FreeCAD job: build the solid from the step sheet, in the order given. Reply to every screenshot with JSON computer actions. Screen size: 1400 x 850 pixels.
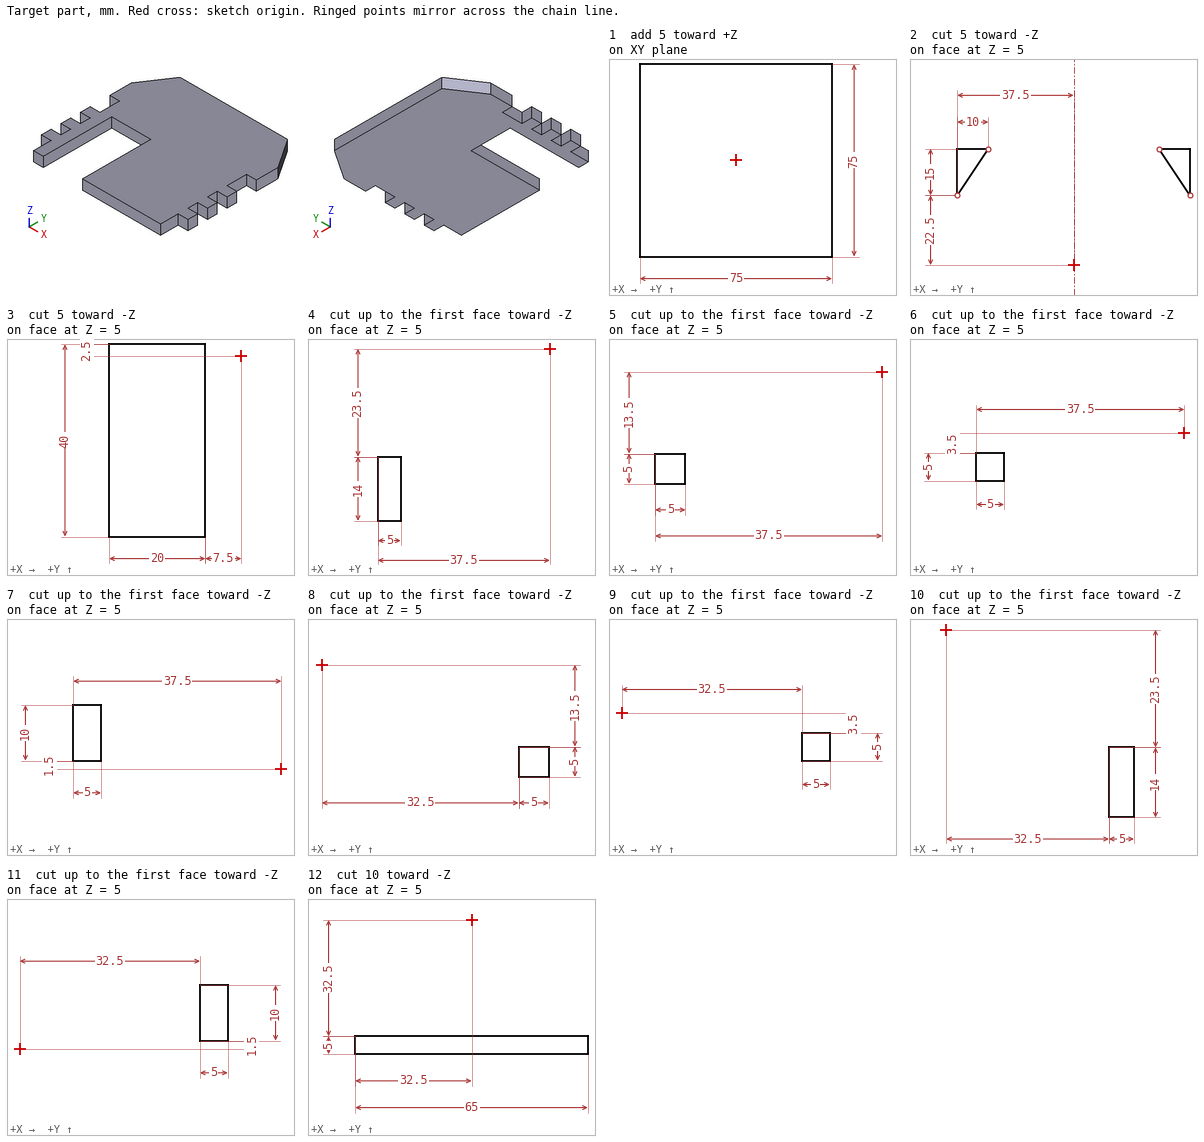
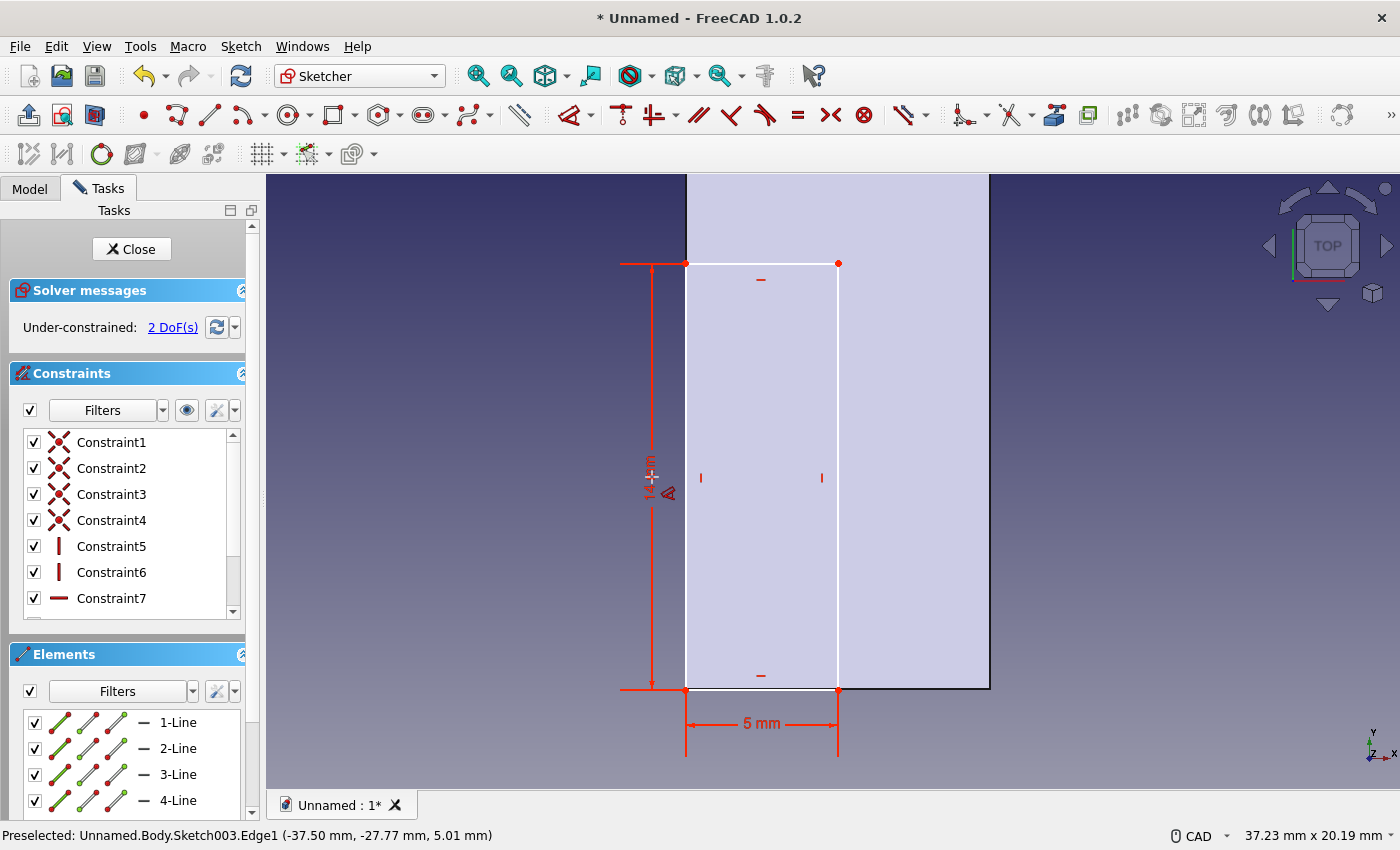
{"action": "left_click", "coordinate": [686, 264]}
{"action": "left_click", "coordinate": [960, 298]}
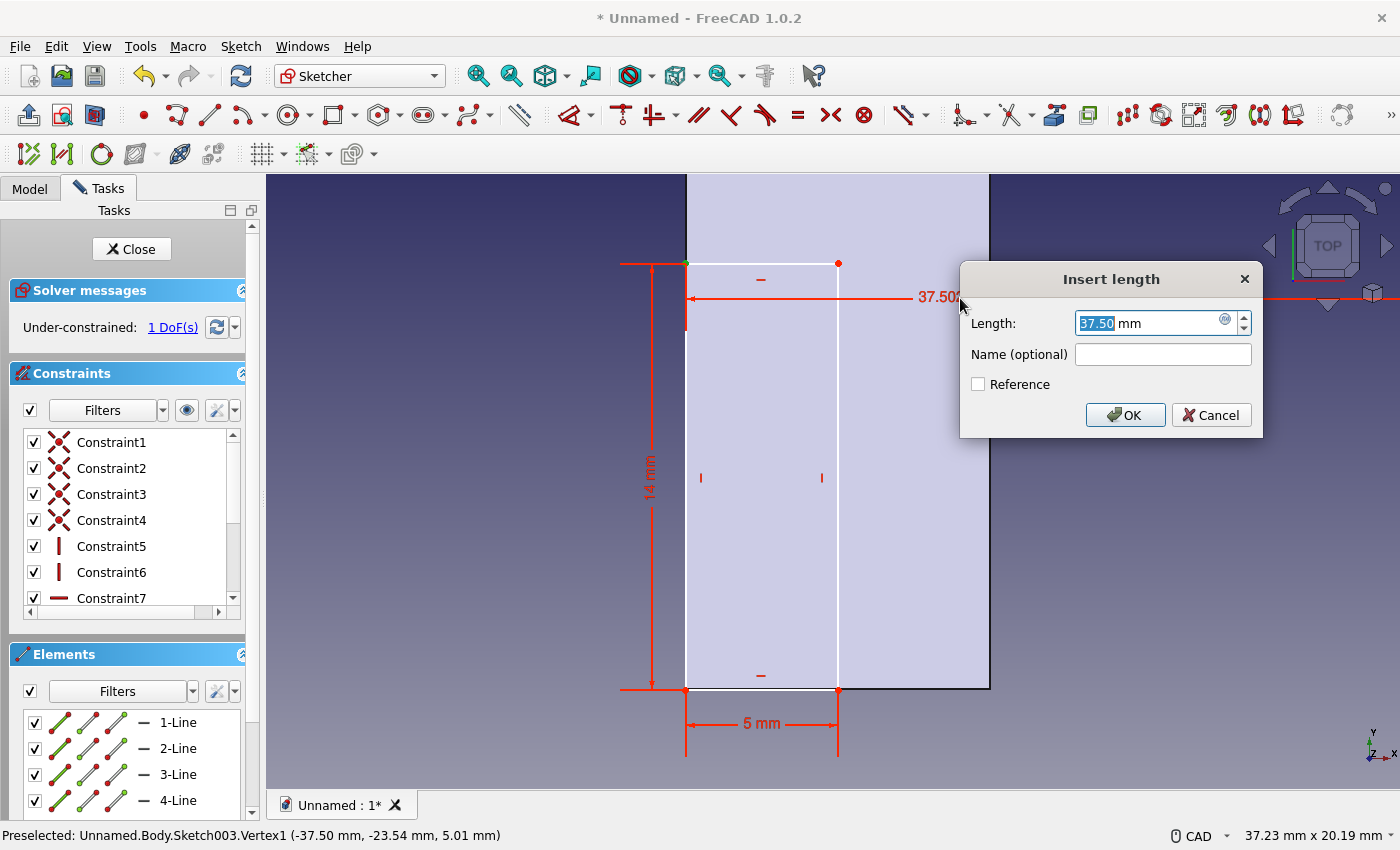
{"action": "type", "text": "37.5"}
{"action": "key", "text": "Return"}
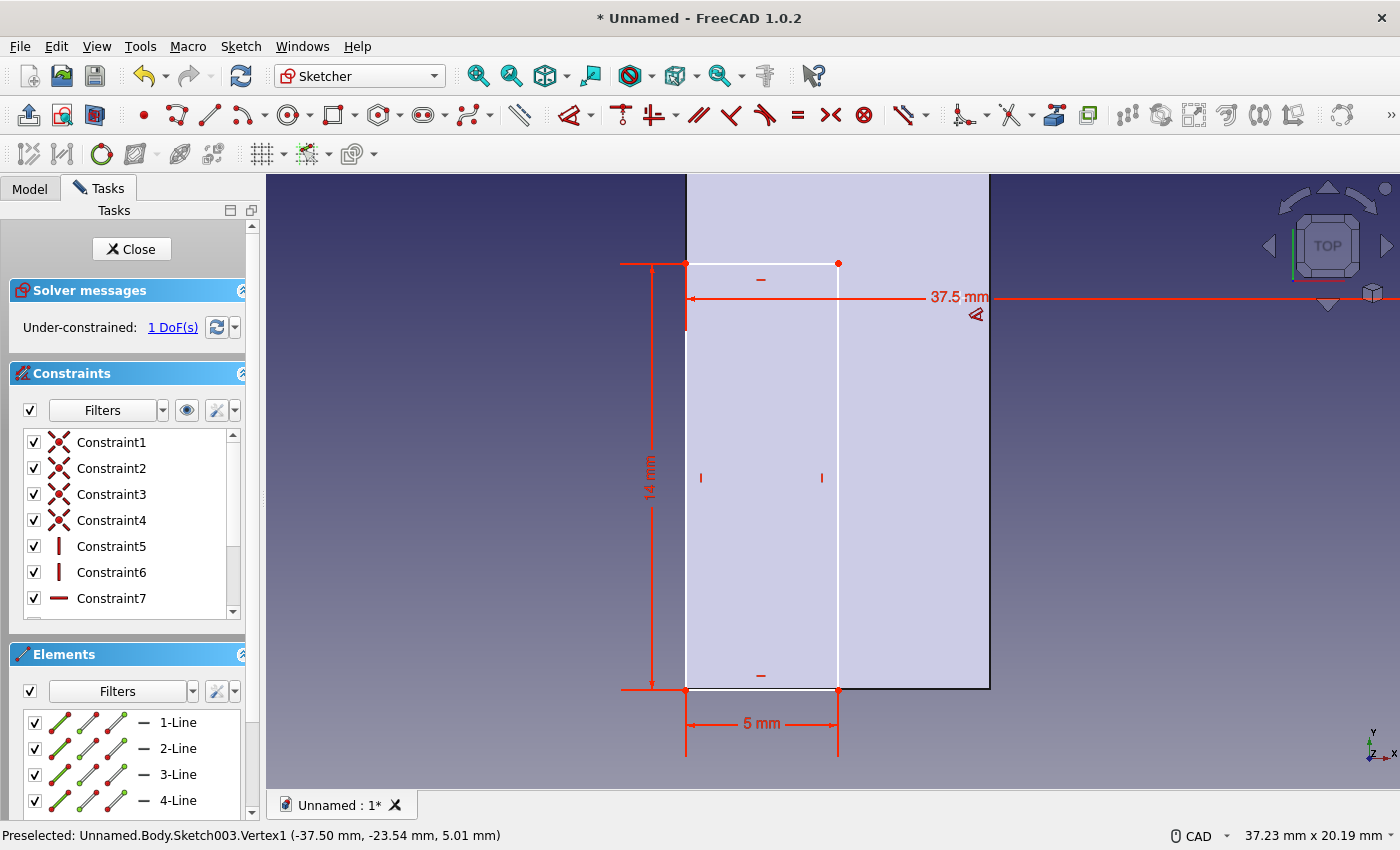
{"action": "left_click", "coordinate": [686, 264]}
{"action": "left_click", "coordinate": [652, 233]}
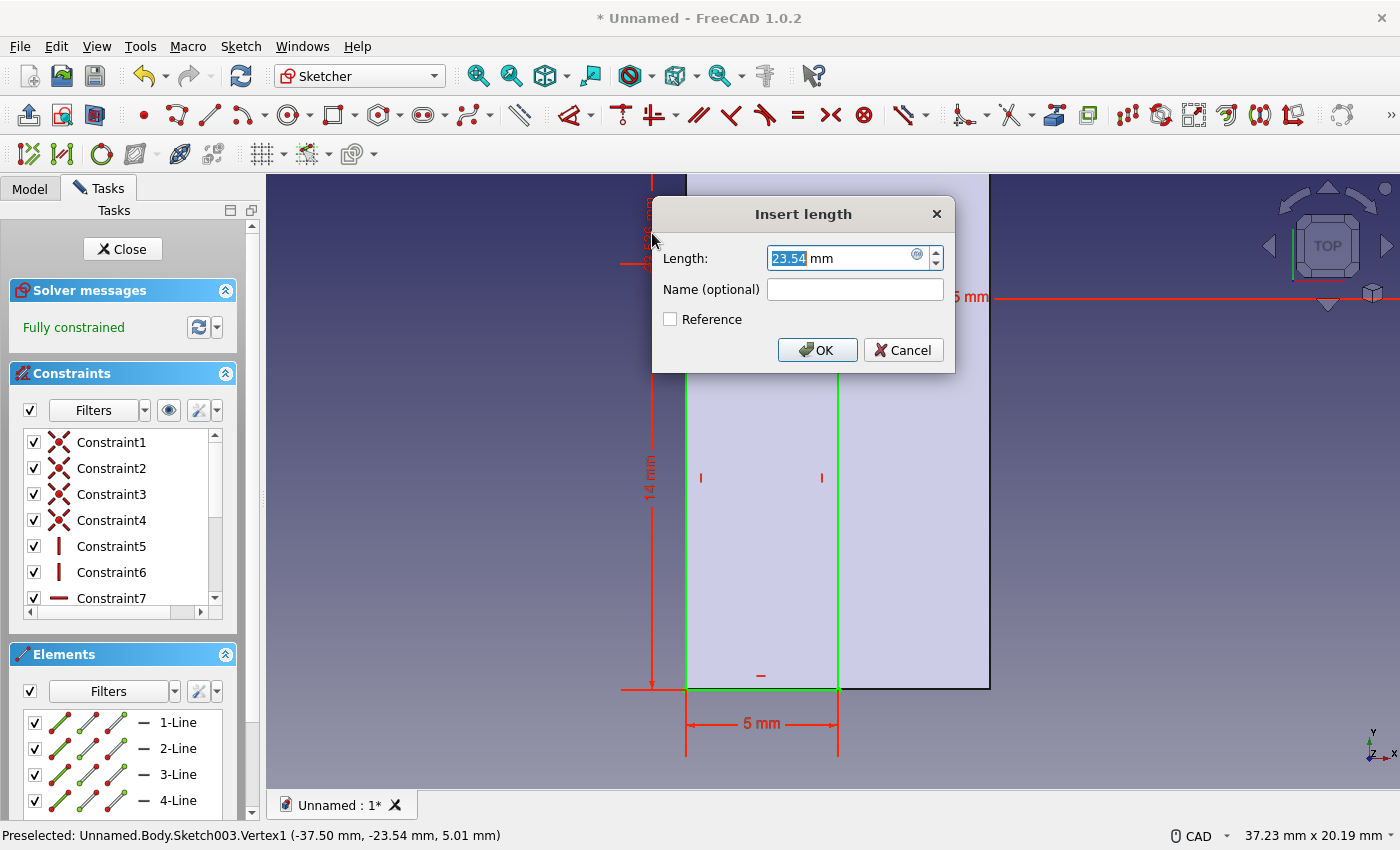
{"action": "type", "text": "23.5"}
{"action": "key", "text": "Return"}
{"action": "key", "text": "Escape"}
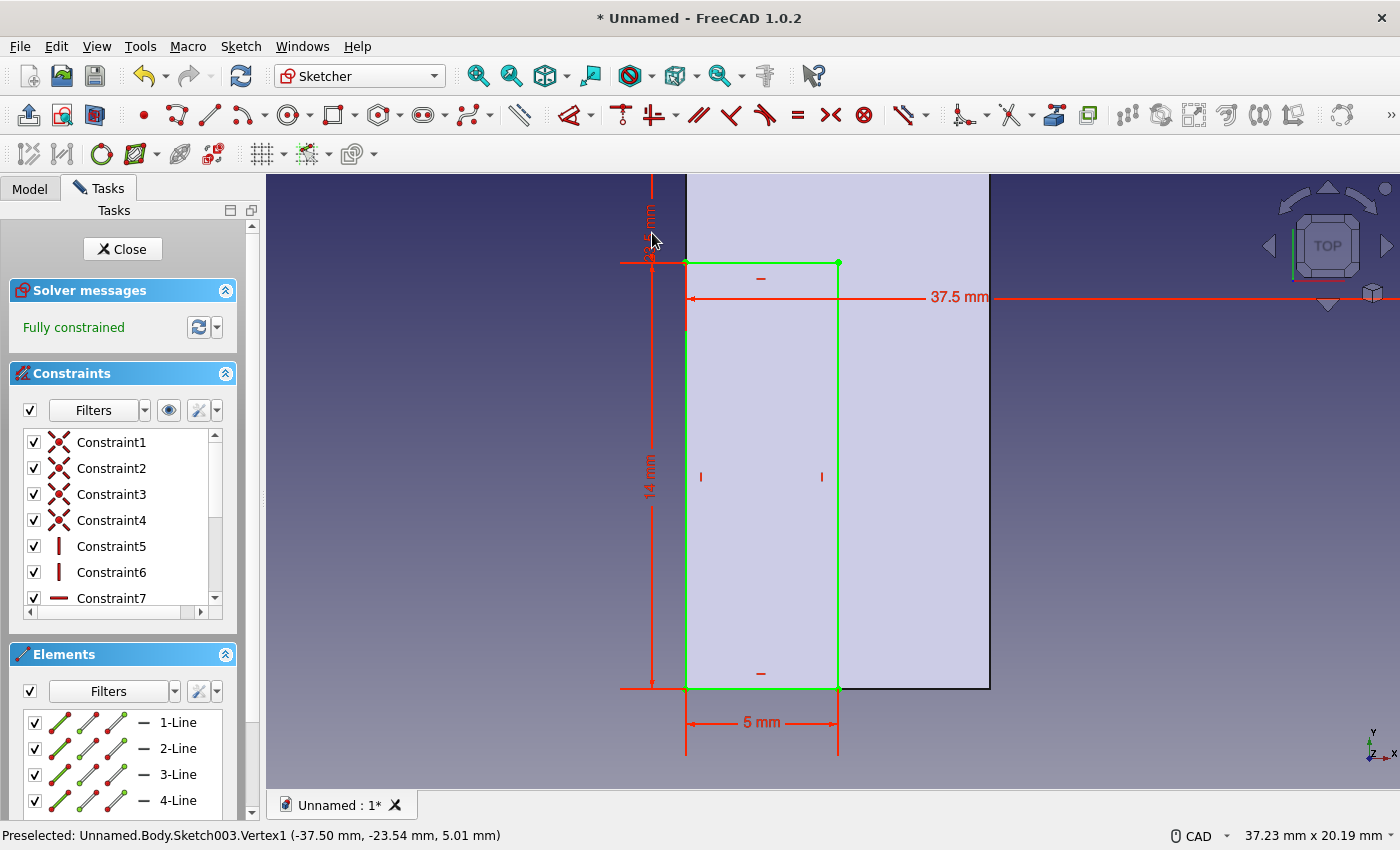
{"action": "left_click", "coordinate": [123, 249]}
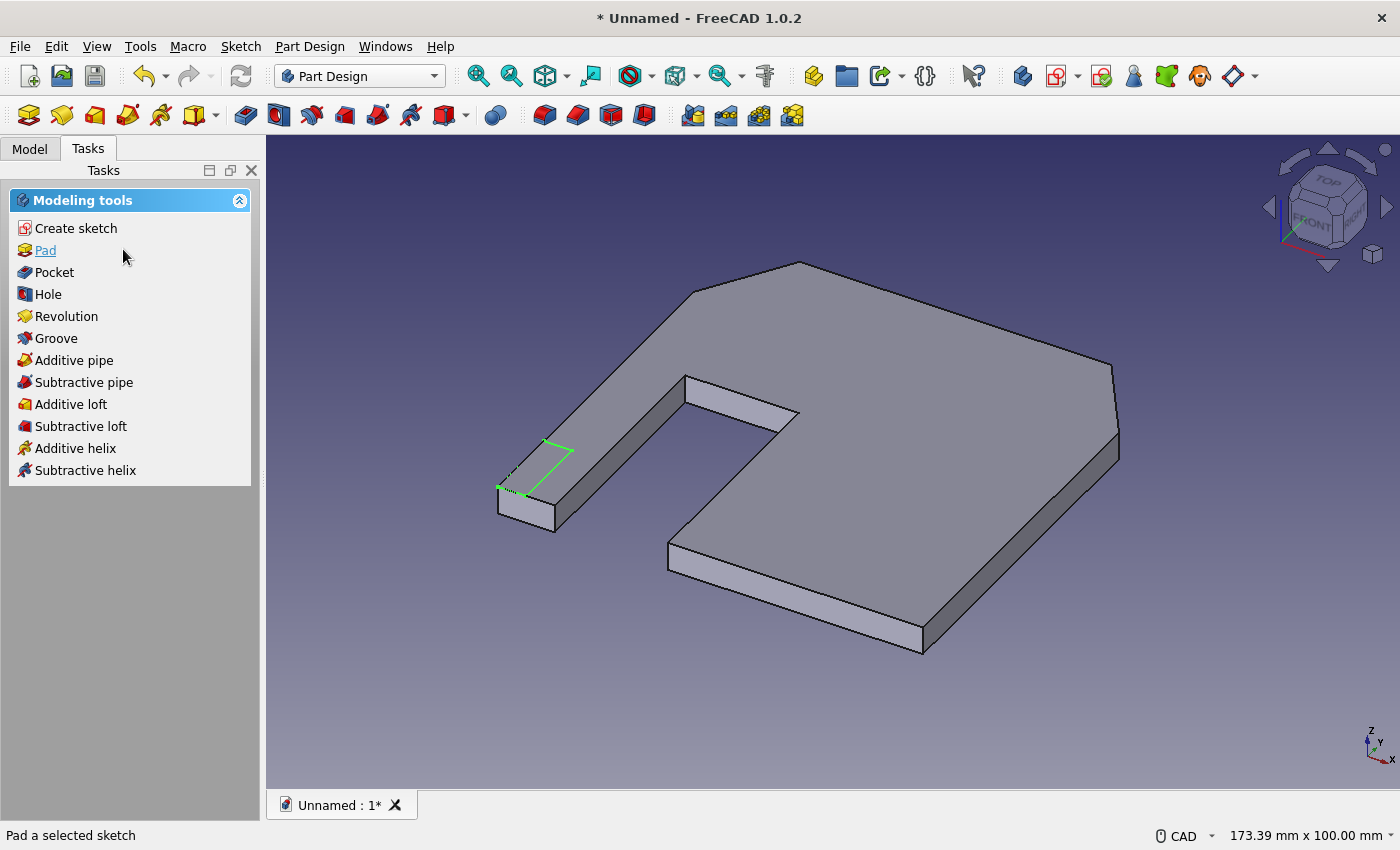
{"action": "left_click", "coordinate": [246, 116]}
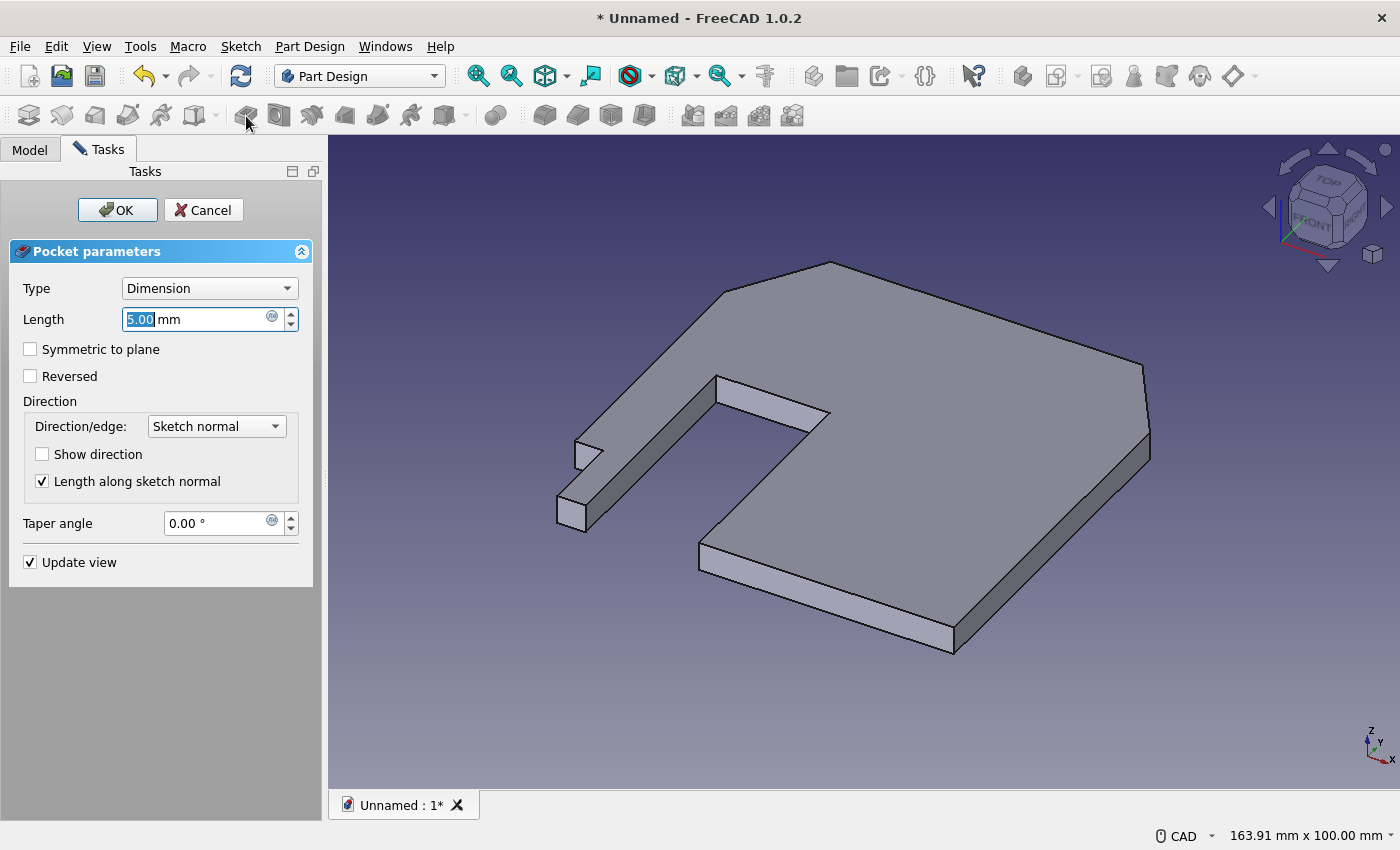
{"action": "left_click", "coordinate": [210, 288]}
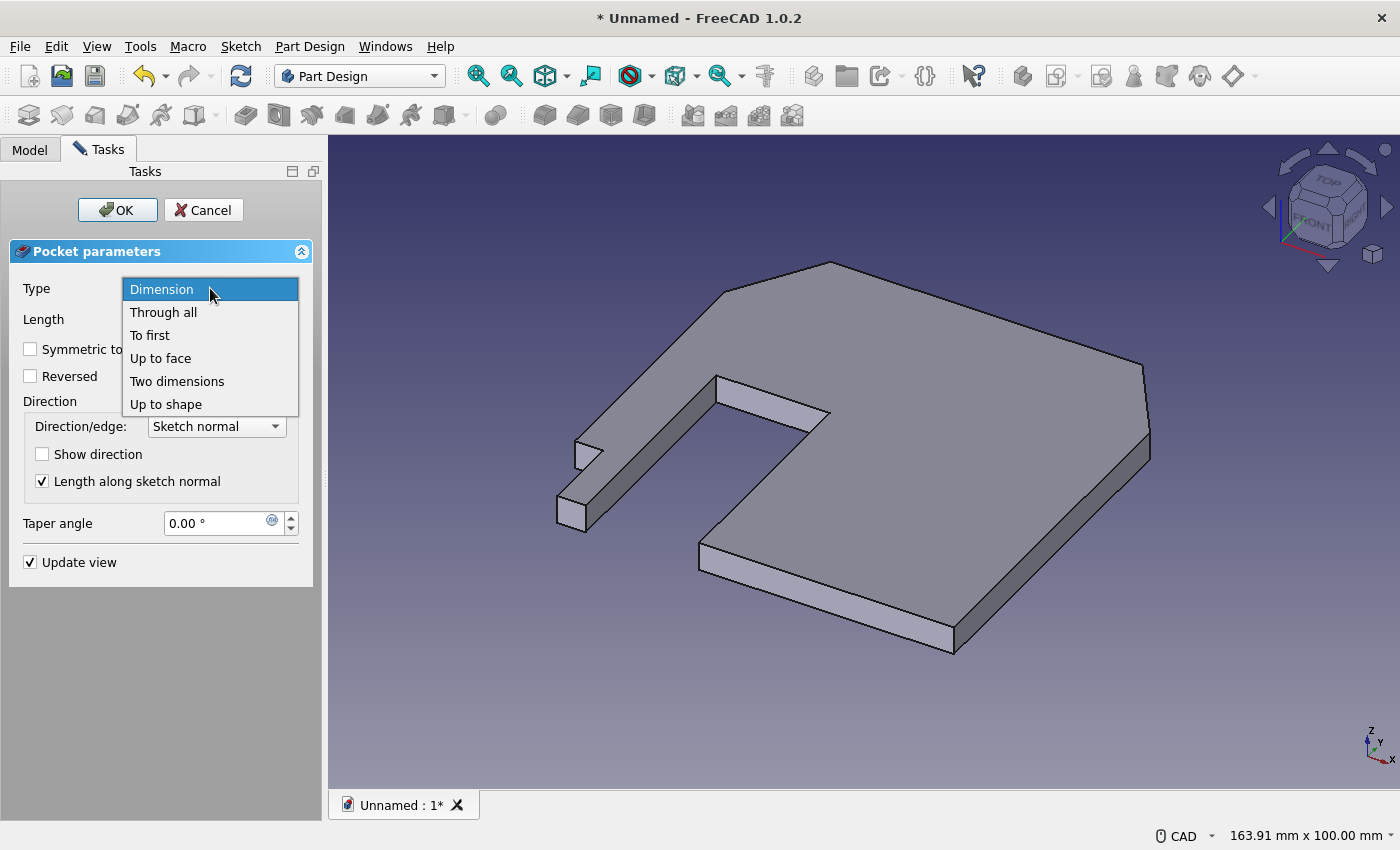
{"action": "left_click", "coordinate": [208, 336]}